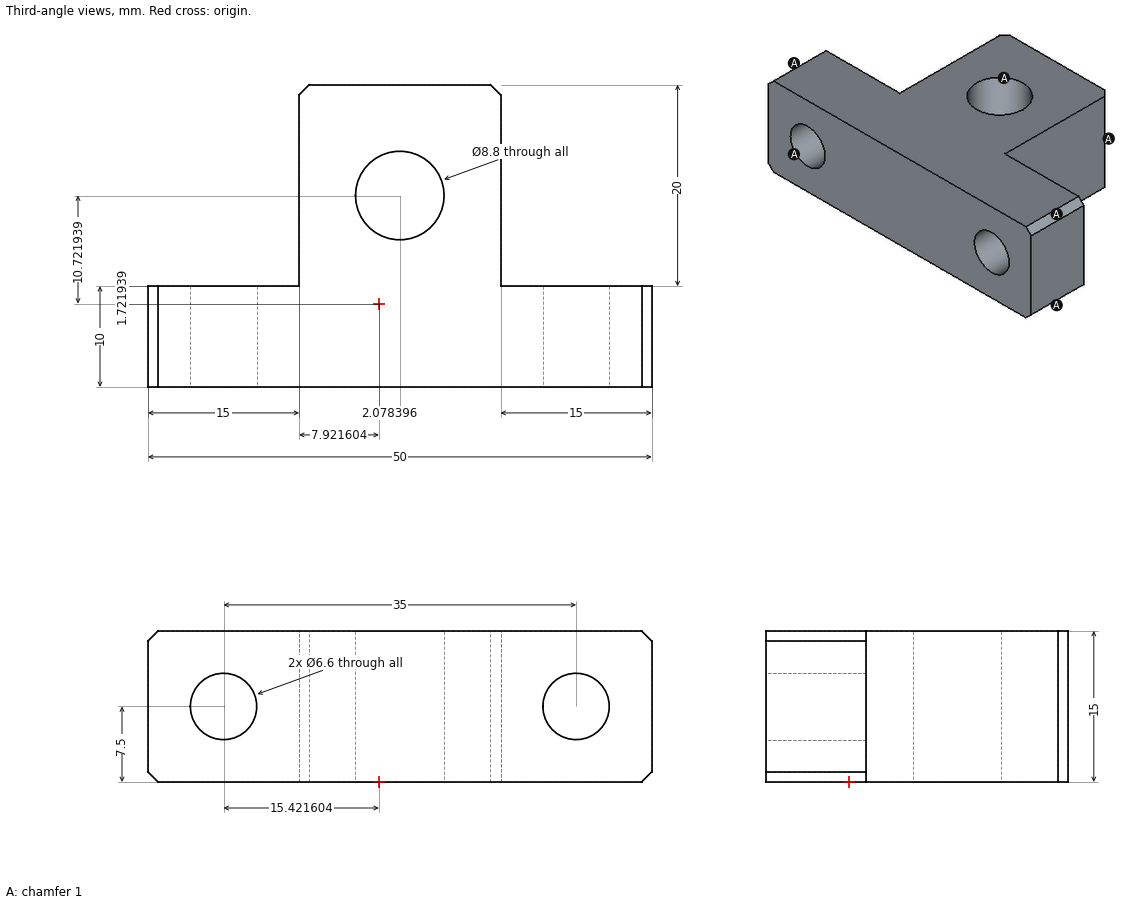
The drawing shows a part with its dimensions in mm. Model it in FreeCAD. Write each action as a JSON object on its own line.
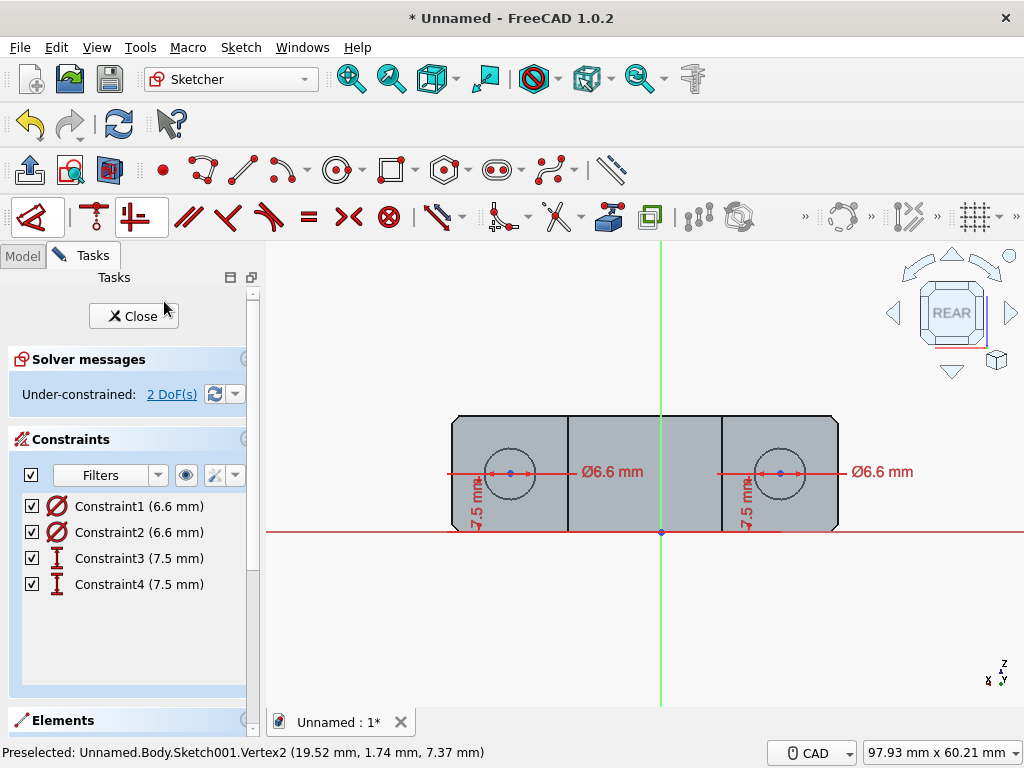
{"action": "left_click", "coordinate": [780, 474]}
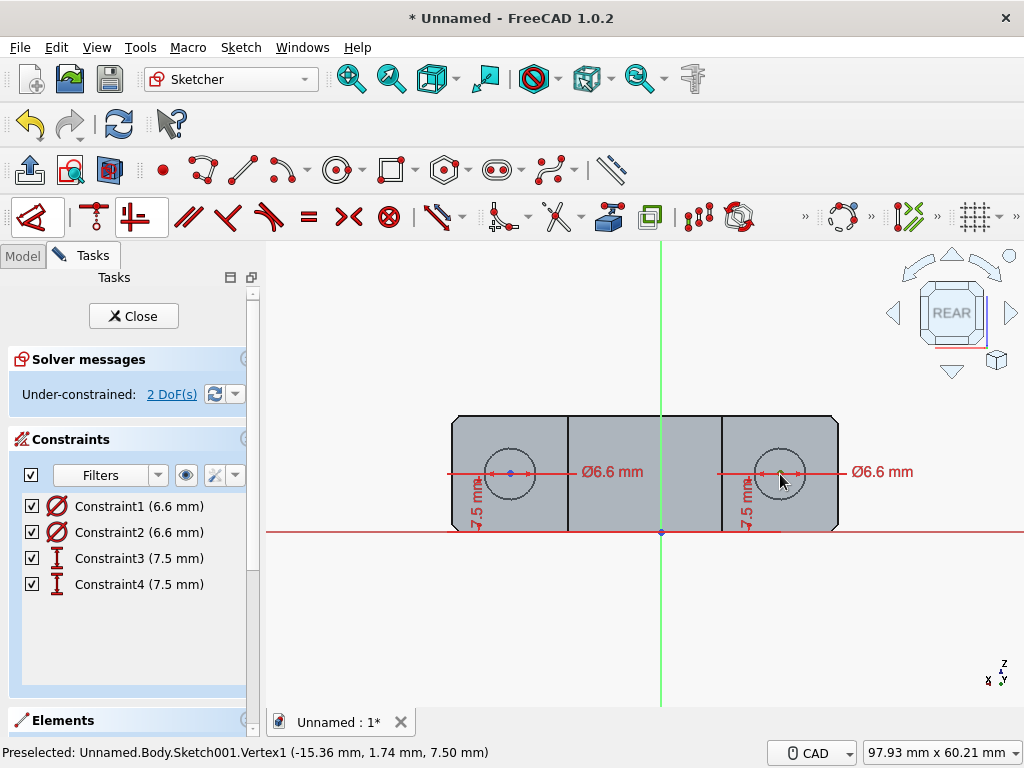
{"action": "left_click", "coordinate": [510, 474]}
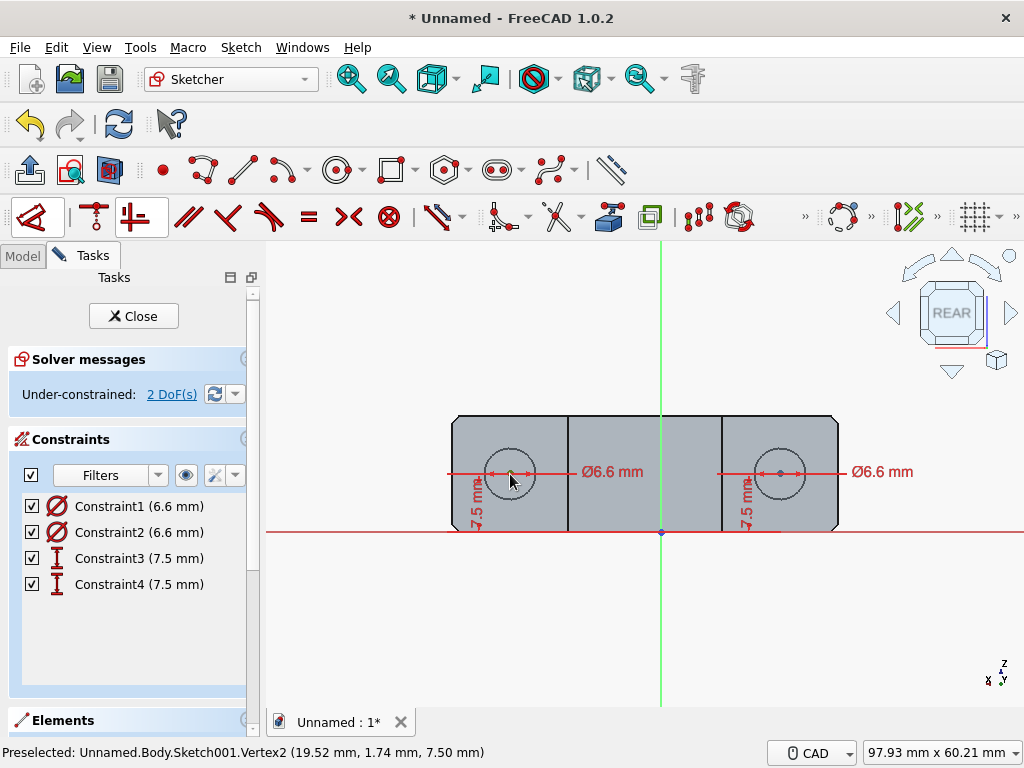
{"action": "key", "text": "l"}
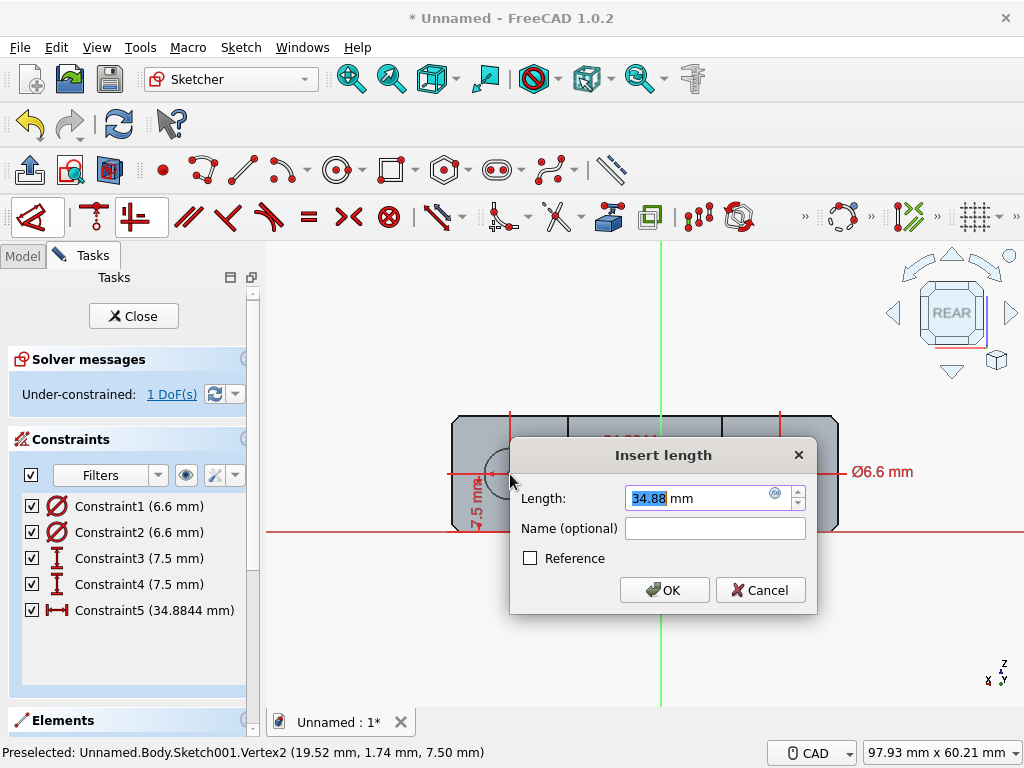
{"action": "type", "text": "35"}
{"action": "key", "text": "Return"}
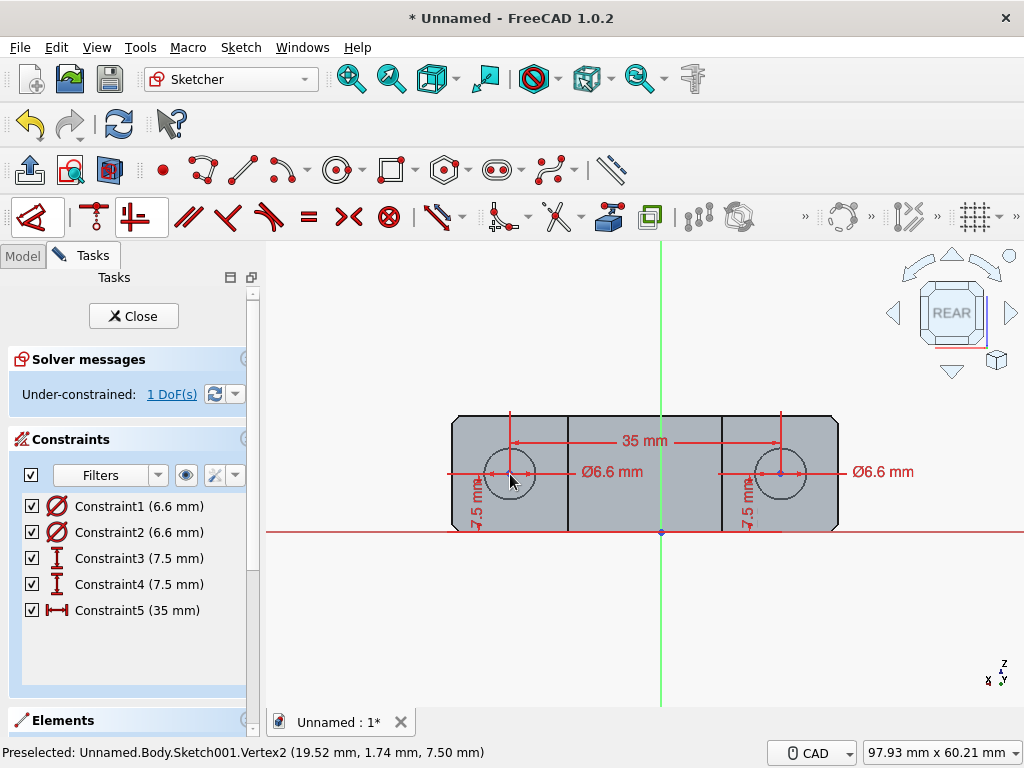
{"action": "left_click", "coordinate": [781, 474]}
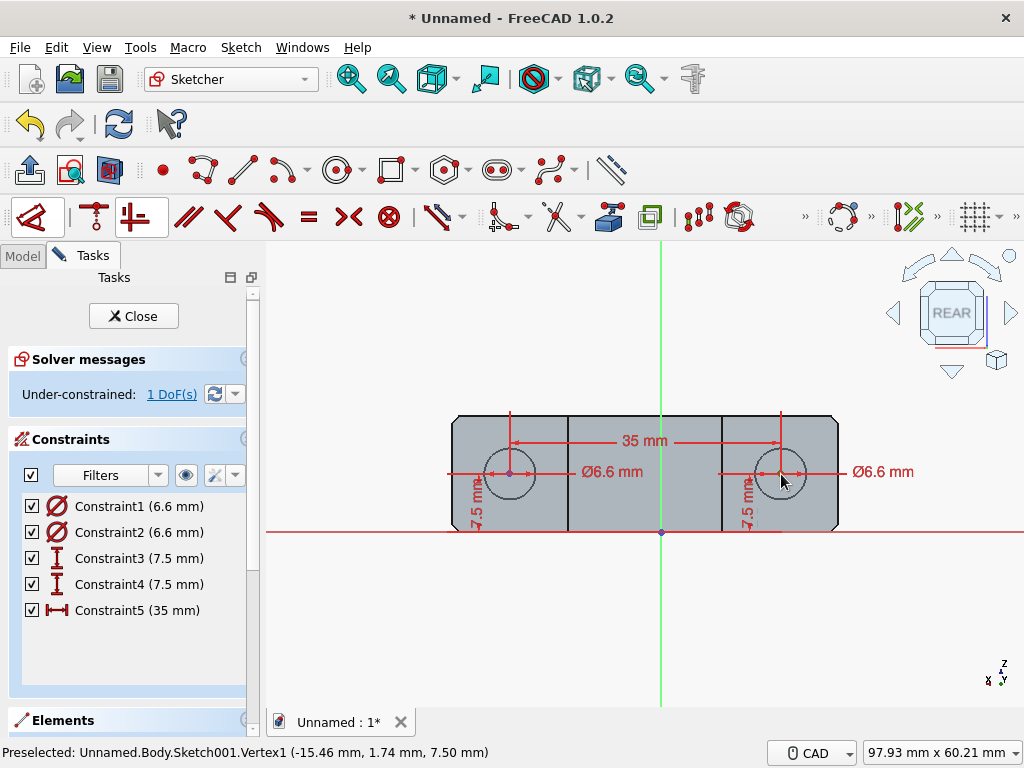
{"action": "key", "text": "l"}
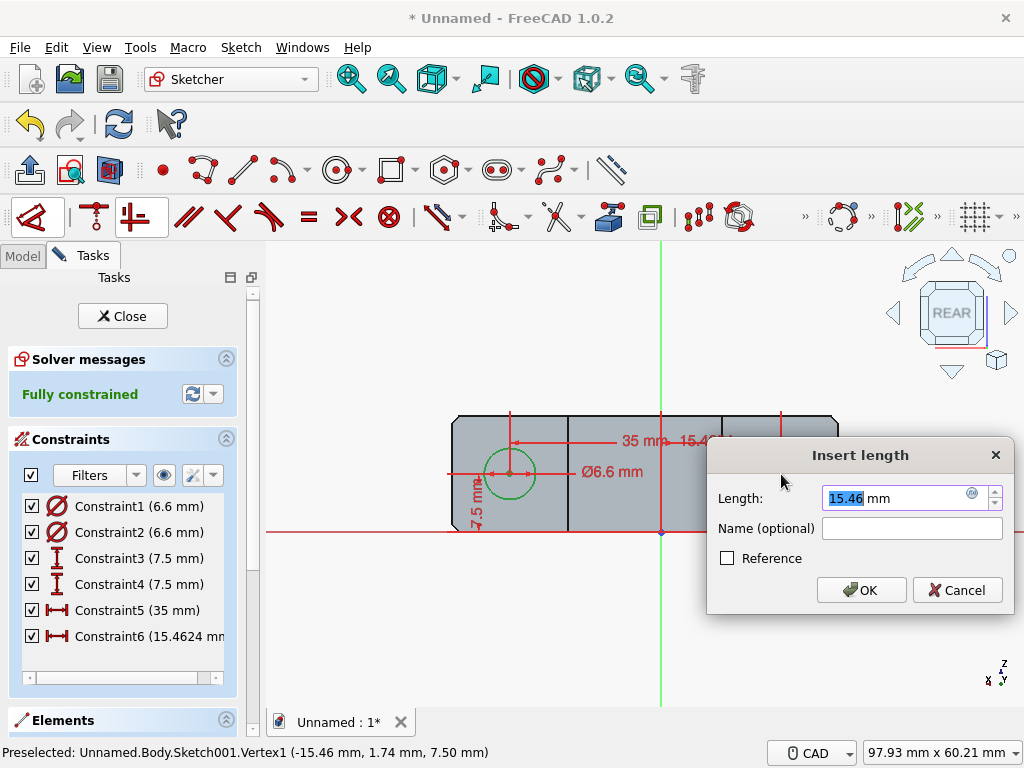
{"action": "type", "text": "15.421604"}
{"action": "key", "text": "Return"}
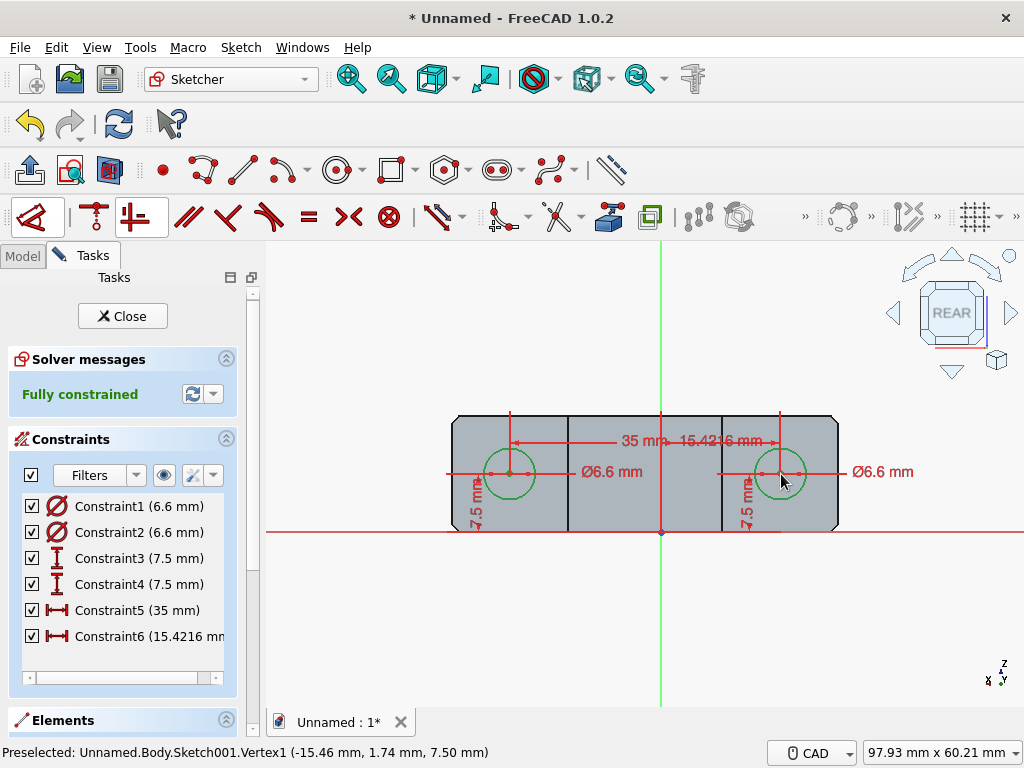
{"action": "left_click", "coordinate": [123, 316]}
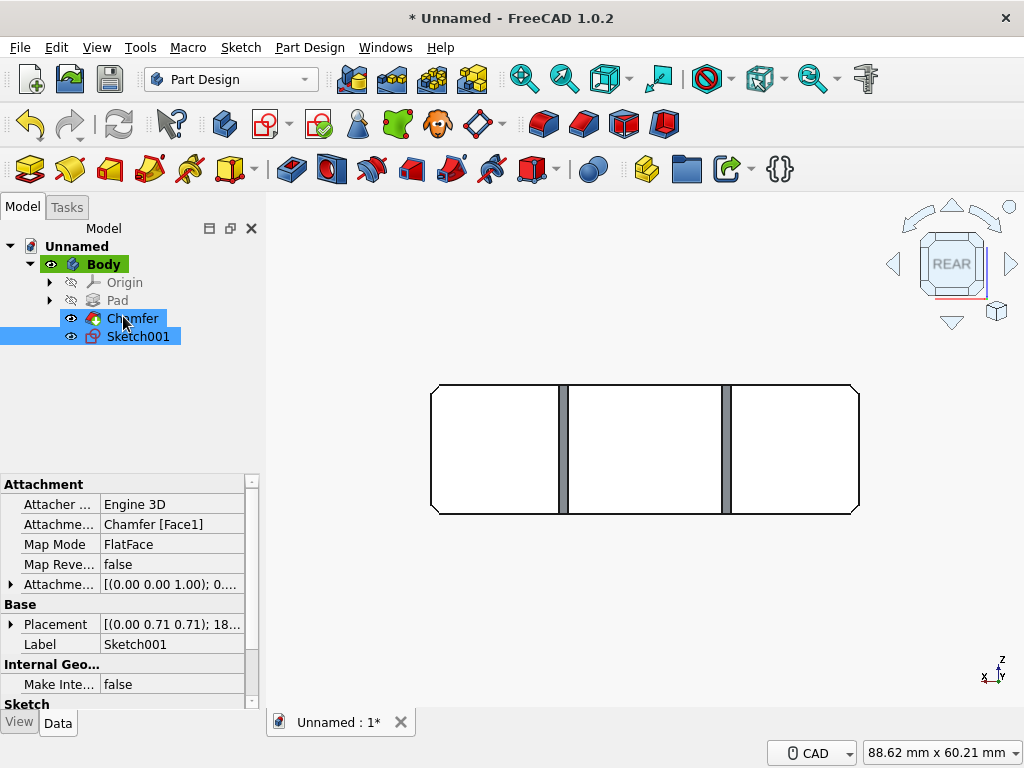
{"action": "left_click", "coordinate": [332, 170]}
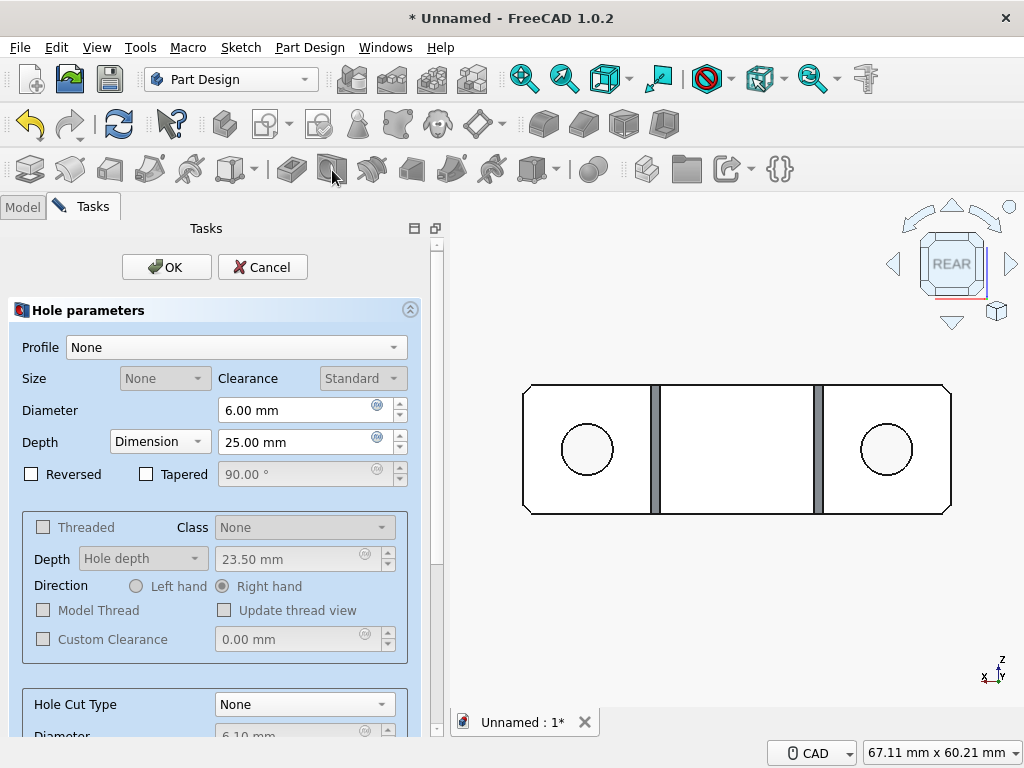
{"action": "triple_click", "coordinate": [305, 410]}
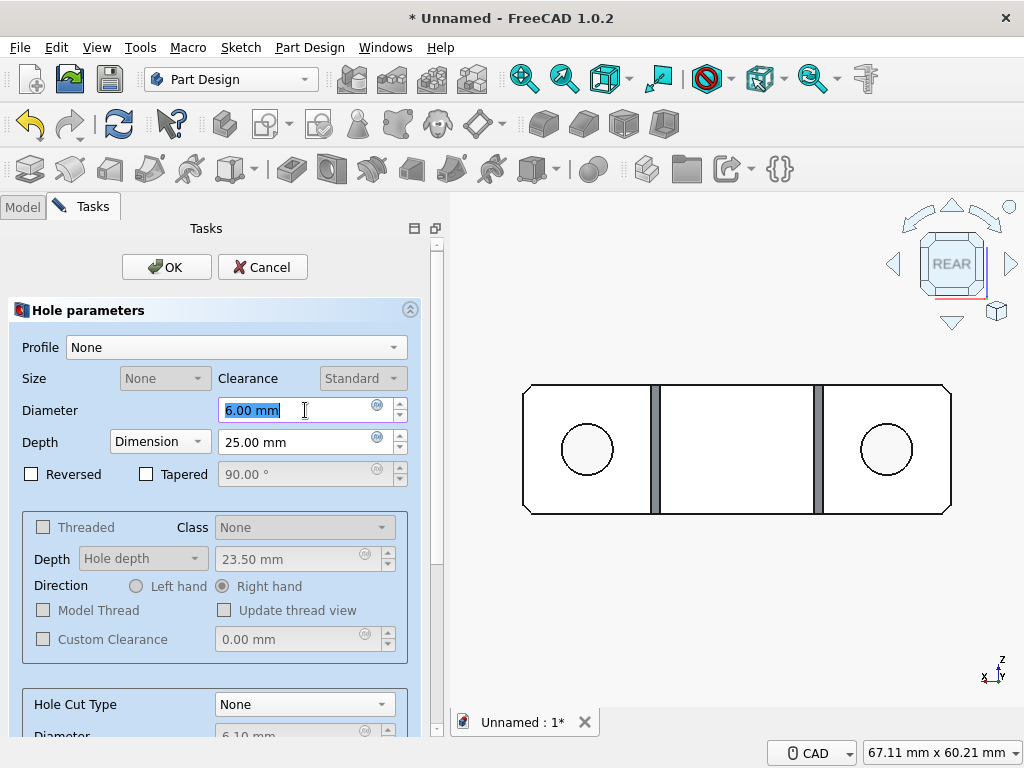
{"action": "type", "text": "6.6"}
{"action": "key", "text": "Tab"}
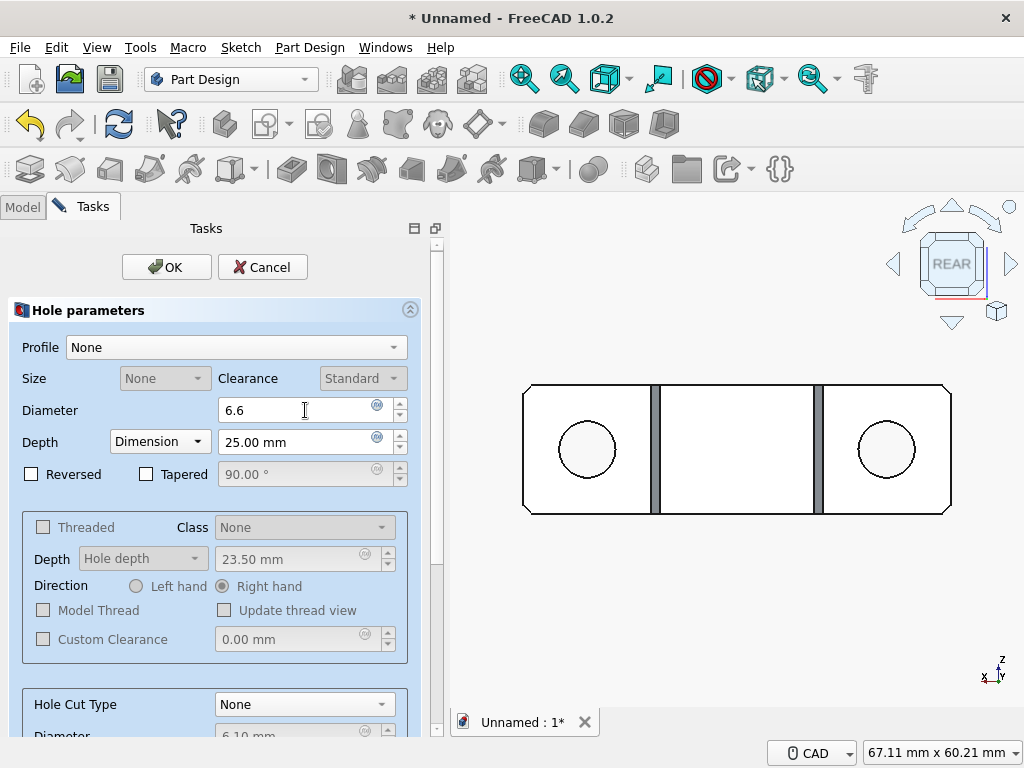
{"action": "left_click", "coordinate": [161, 442]}